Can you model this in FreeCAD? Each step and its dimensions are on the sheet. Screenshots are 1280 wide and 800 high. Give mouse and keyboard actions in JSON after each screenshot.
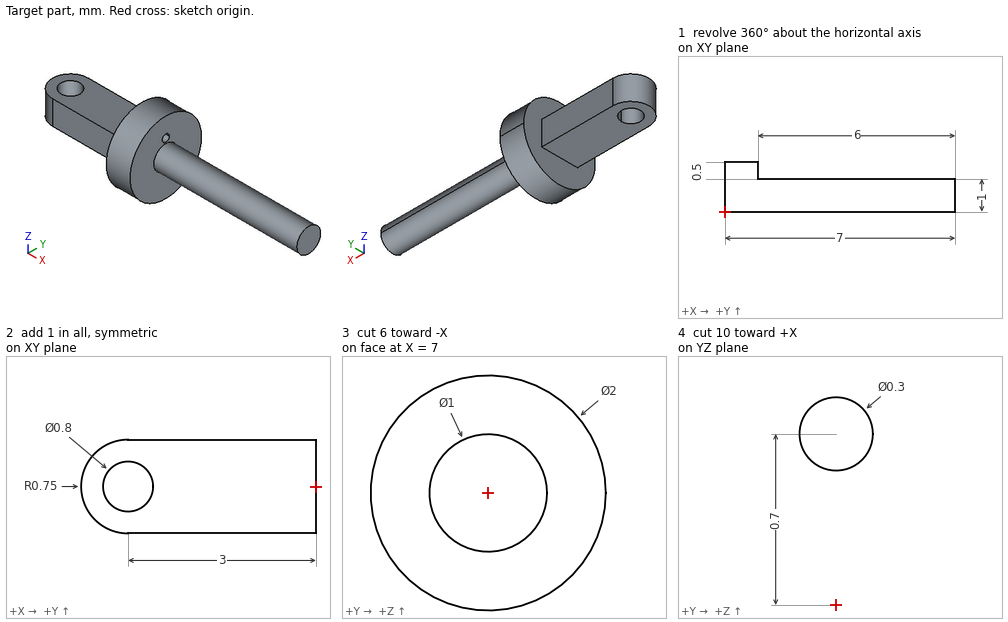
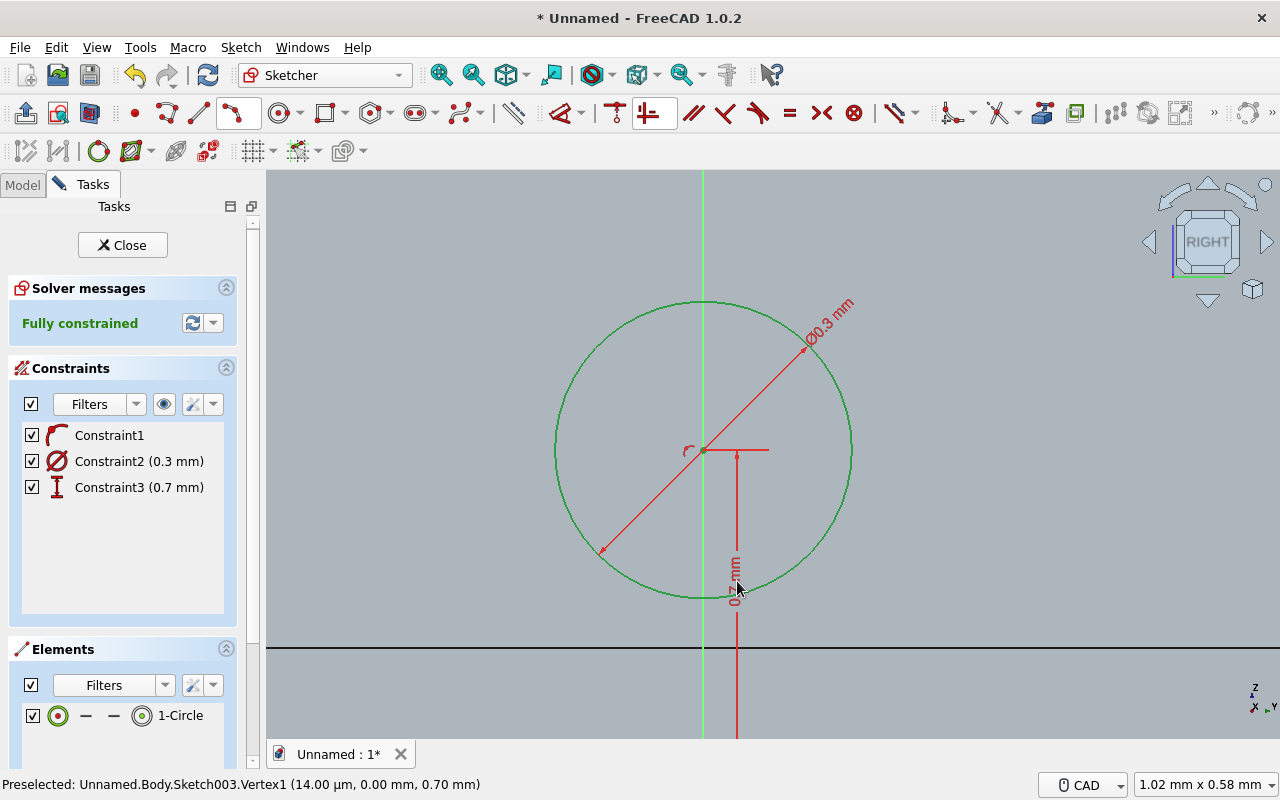
{"action": "left_click", "coordinate": [123, 245]}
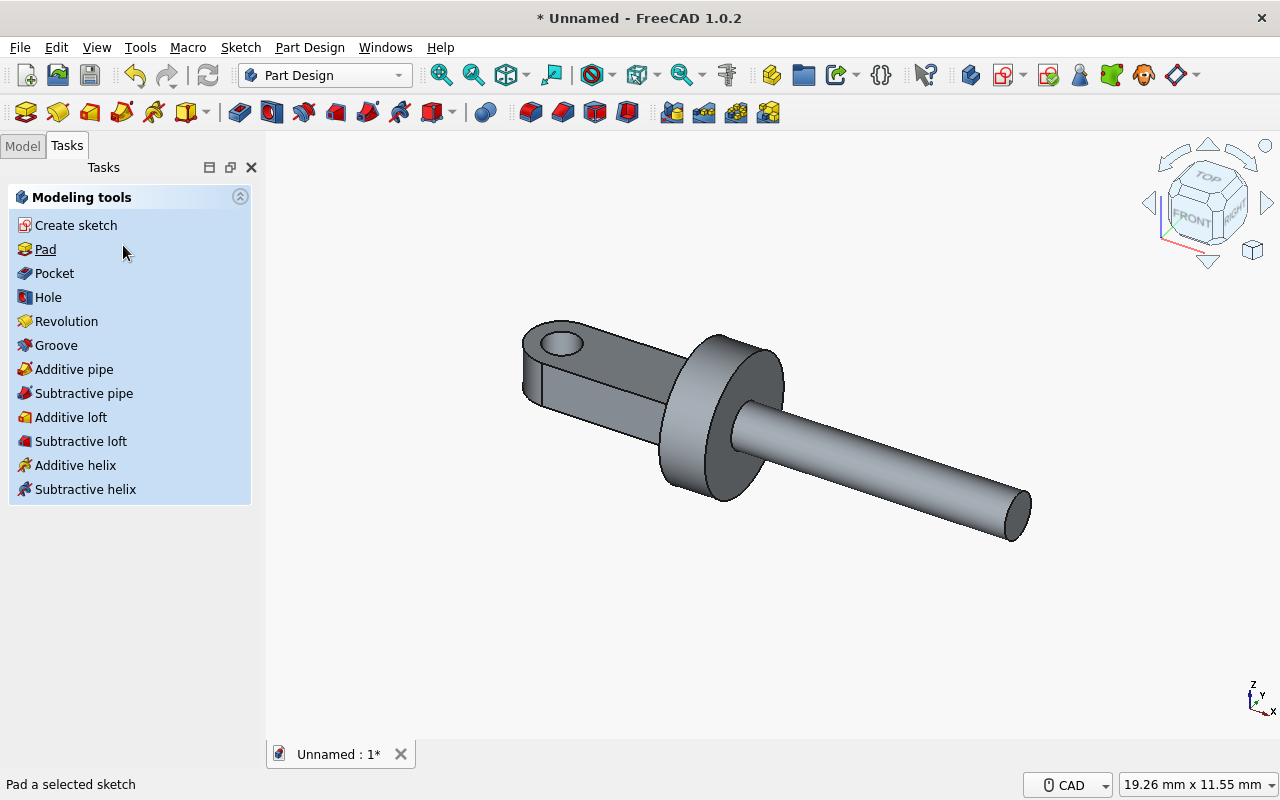
{"action": "left_click", "coordinate": [240, 112]}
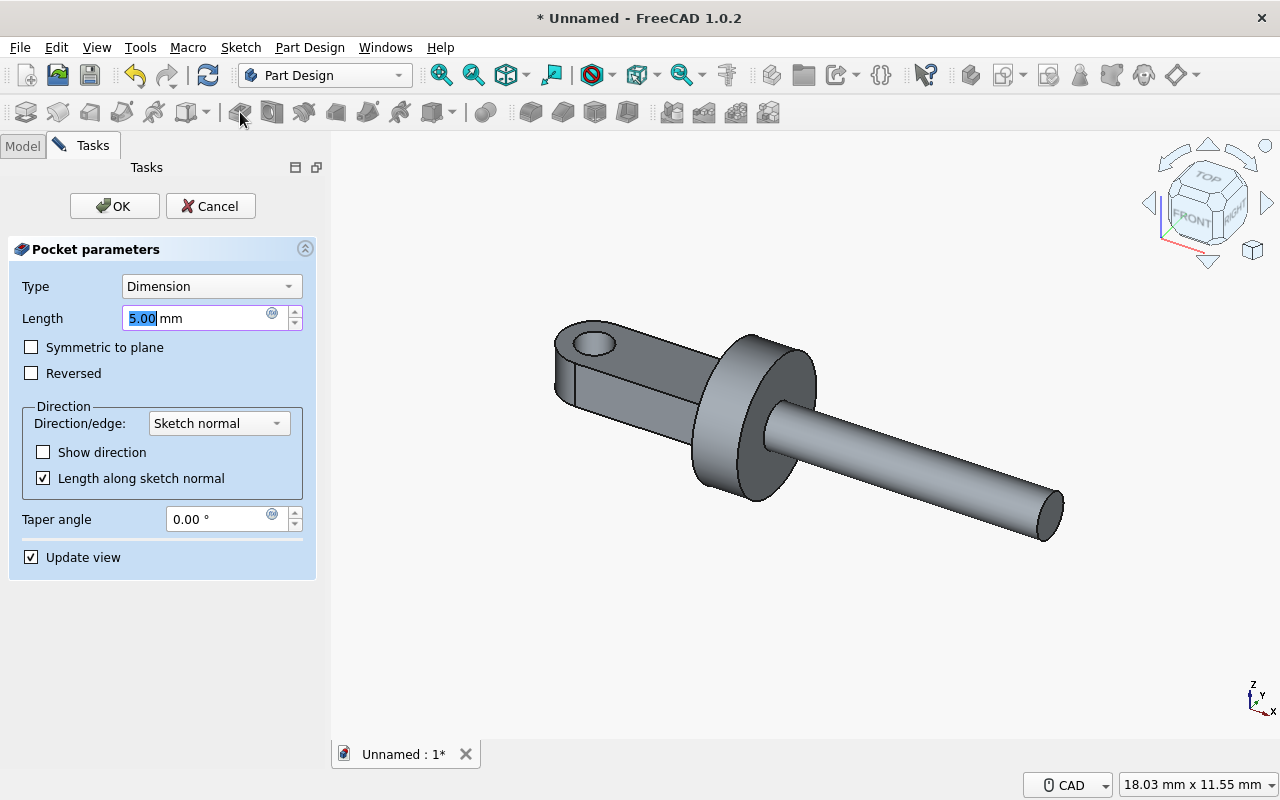
{"action": "type", "text": "10"}
{"action": "key", "text": "Tab"}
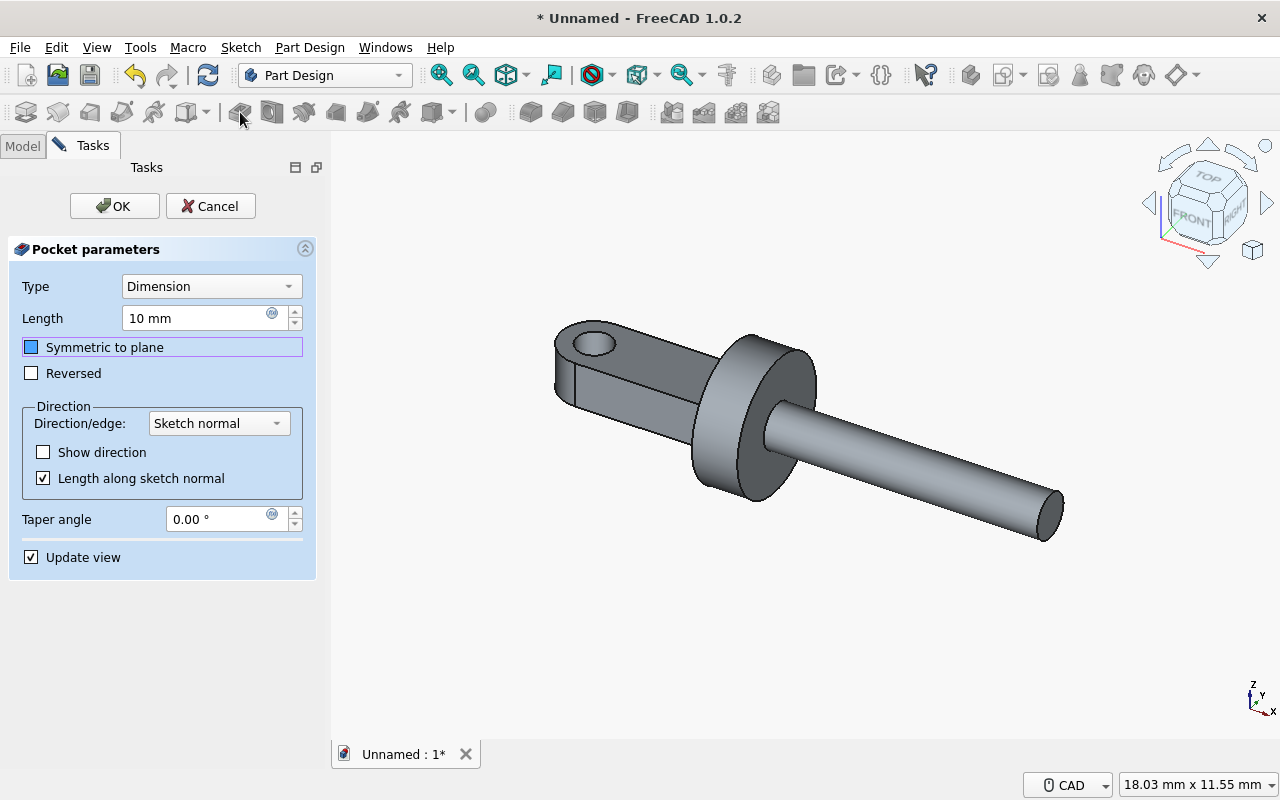
{"action": "left_click", "coordinate": [30, 373]}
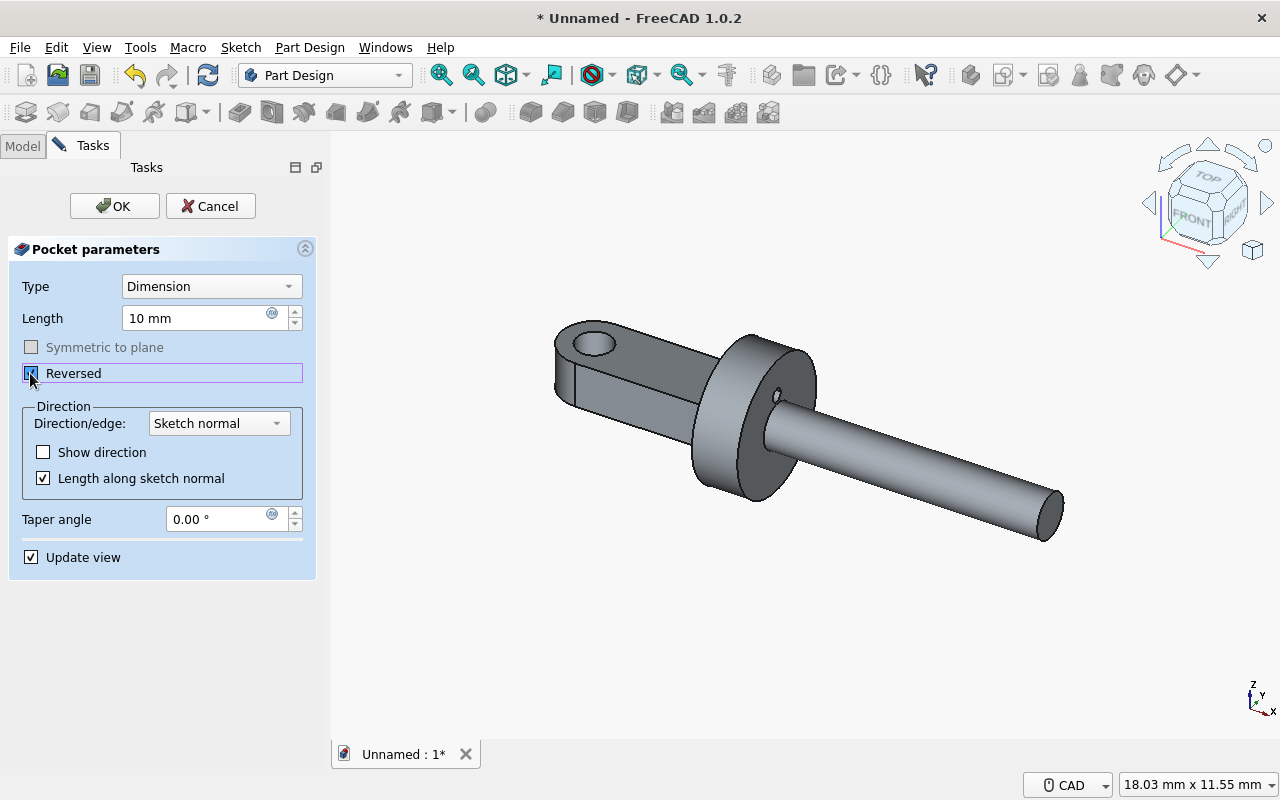
{"action": "left_click", "coordinate": [115, 206]}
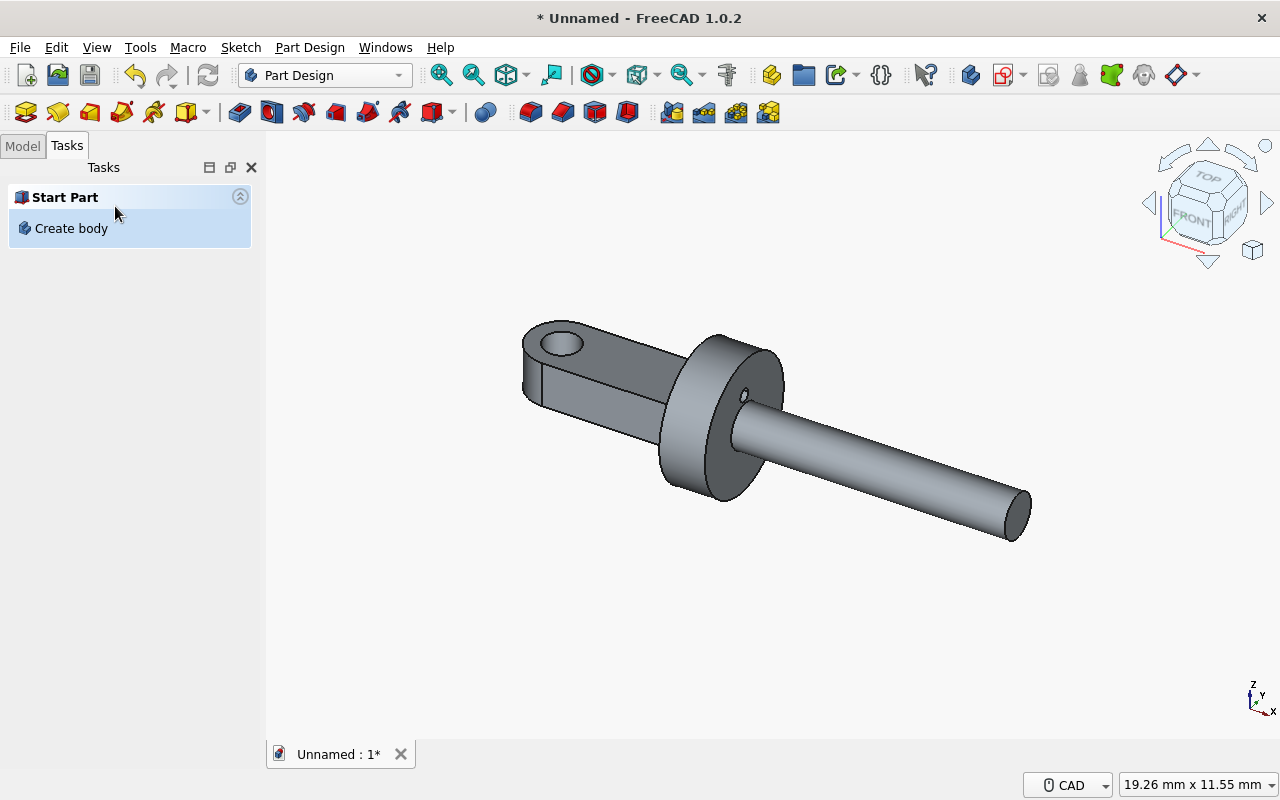
{"action": "key", "text": "0"}